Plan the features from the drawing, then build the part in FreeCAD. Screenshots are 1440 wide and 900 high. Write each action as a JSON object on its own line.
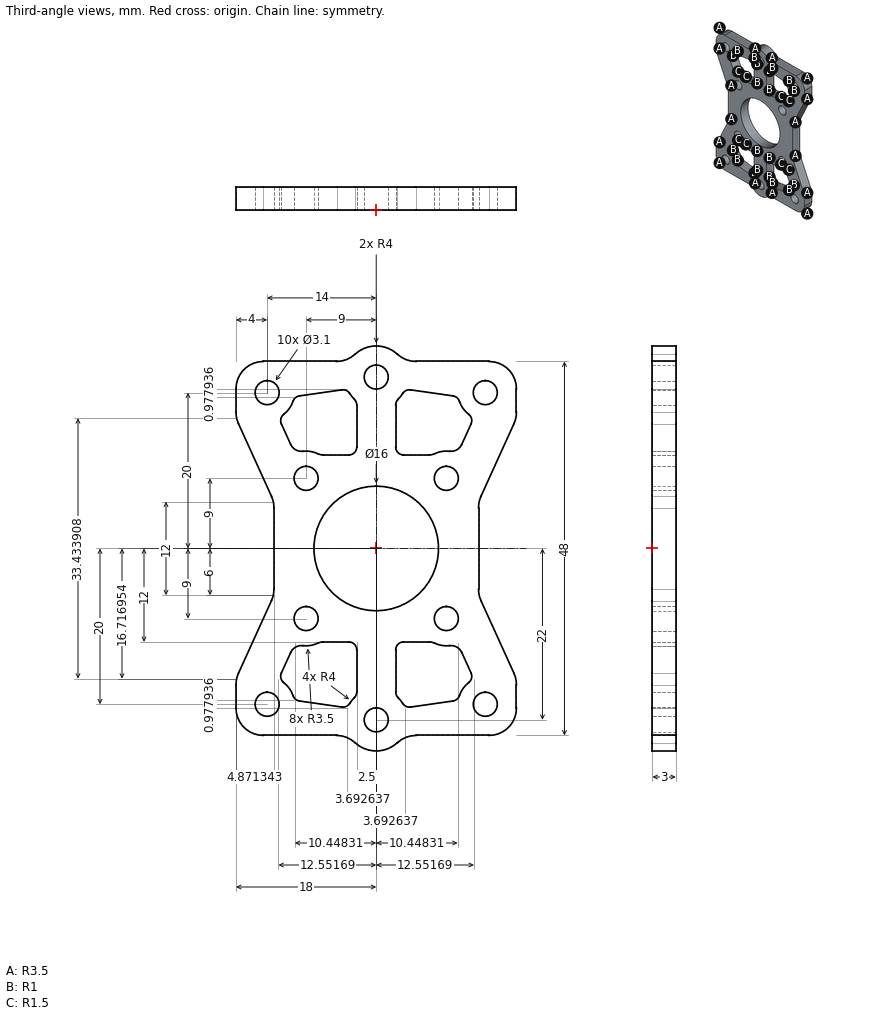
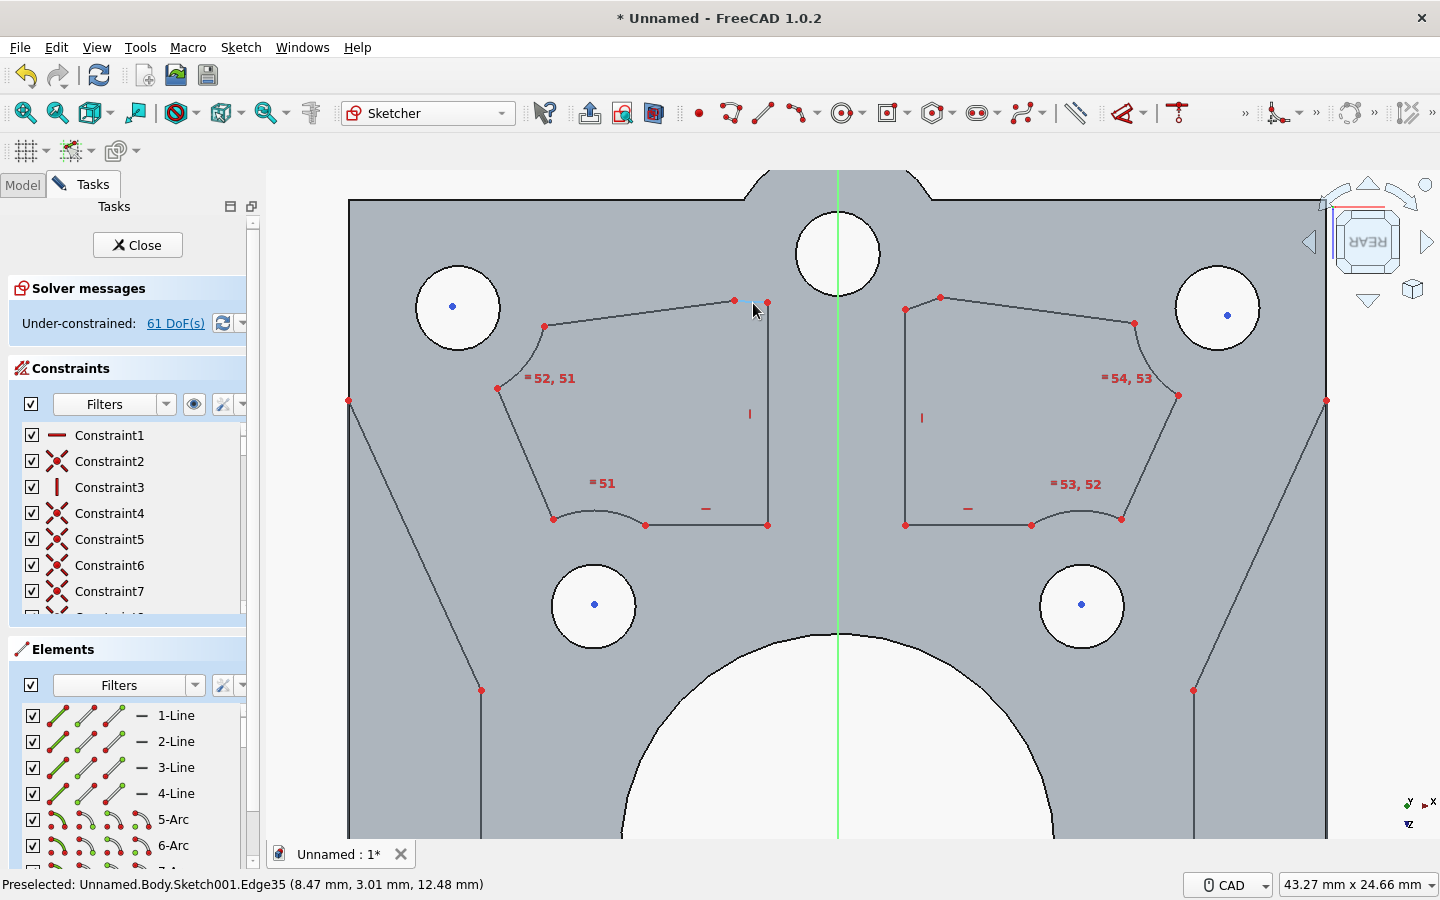
{"action": "left_click", "coordinate": [751, 302]}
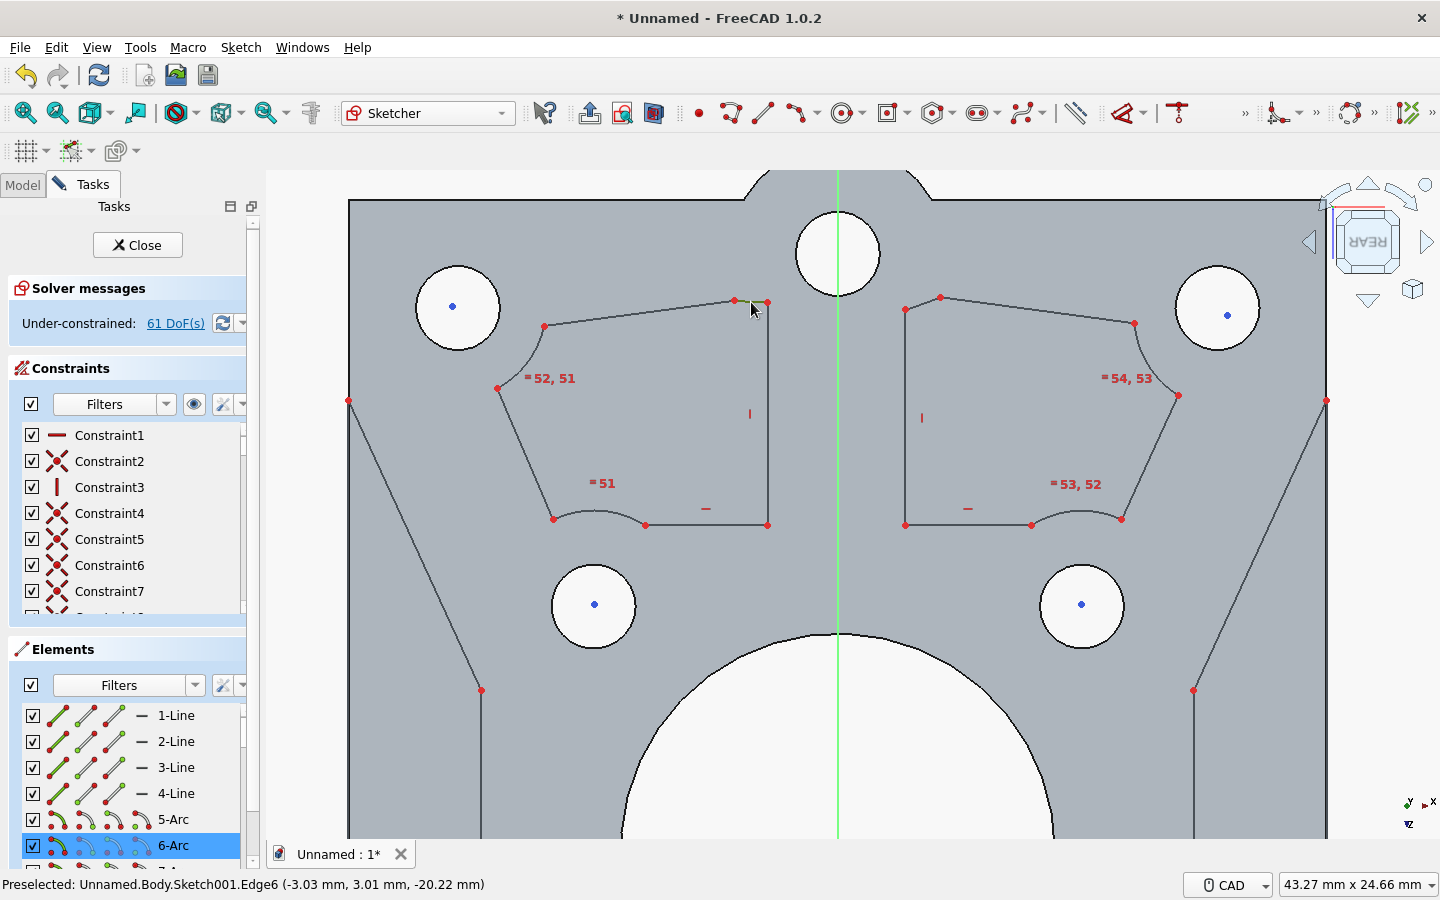
{"action": "scroll", "coordinate": [916, 306], "scroll_direction": "up", "scroll_amount": 2}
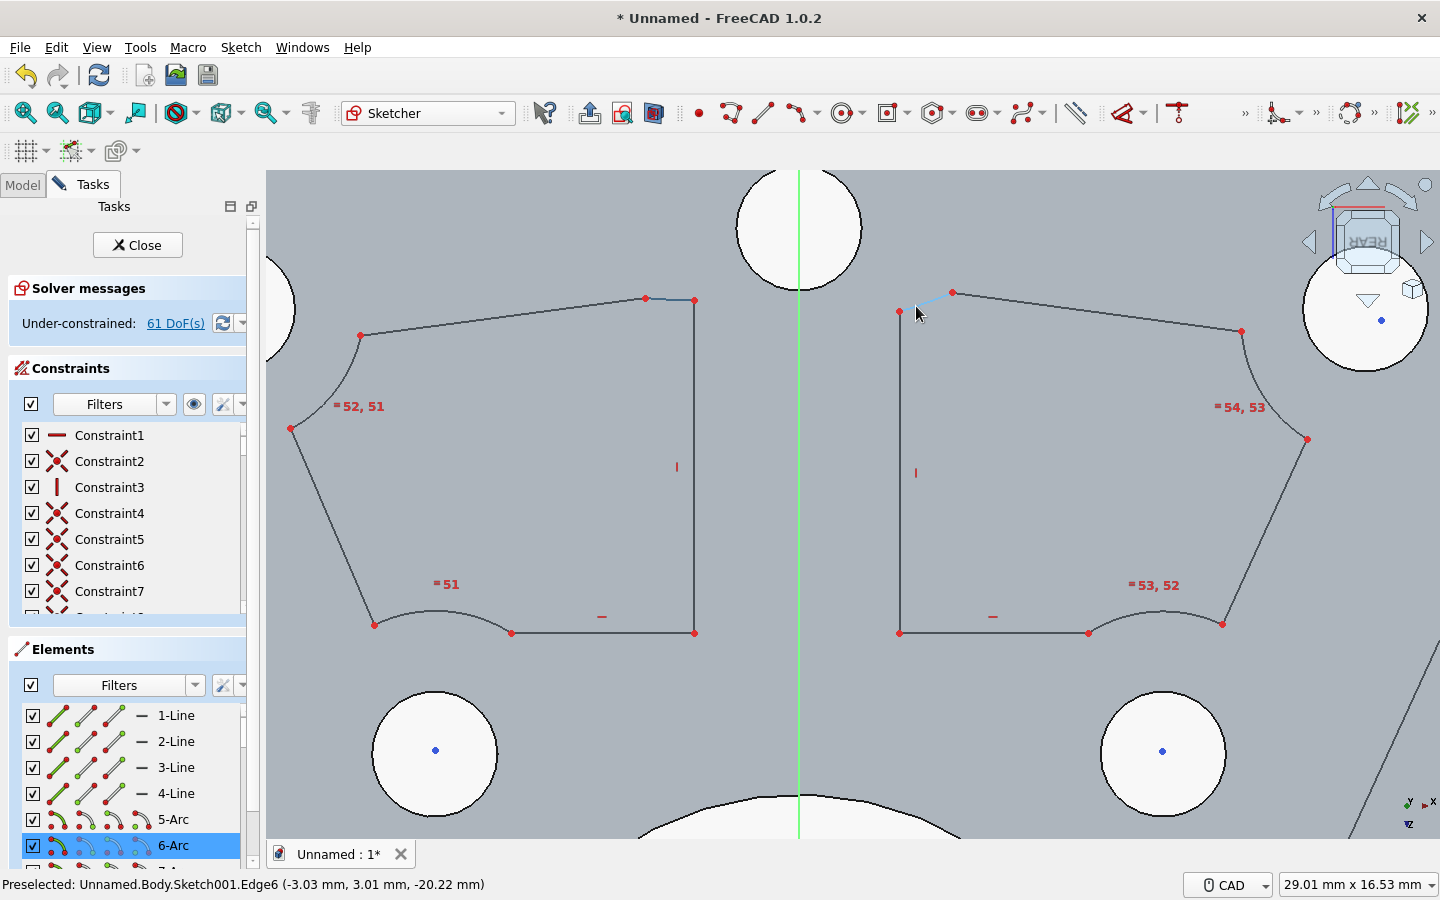
{"action": "left_click", "coordinate": [916, 306]}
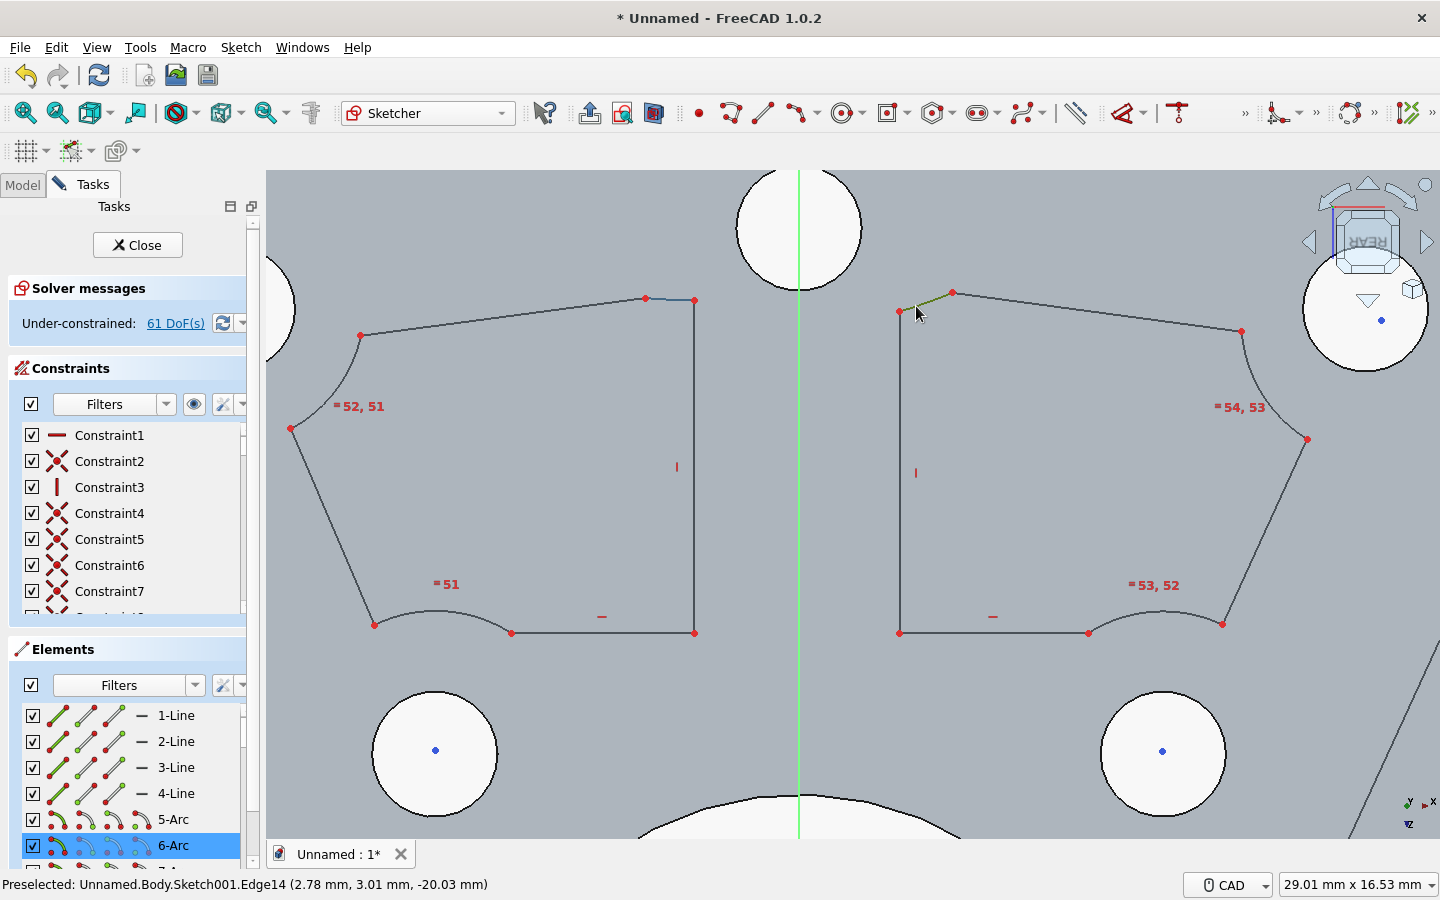
{"action": "scroll", "coordinate": [780, 304], "scroll_direction": "down", "scroll_amount": 7}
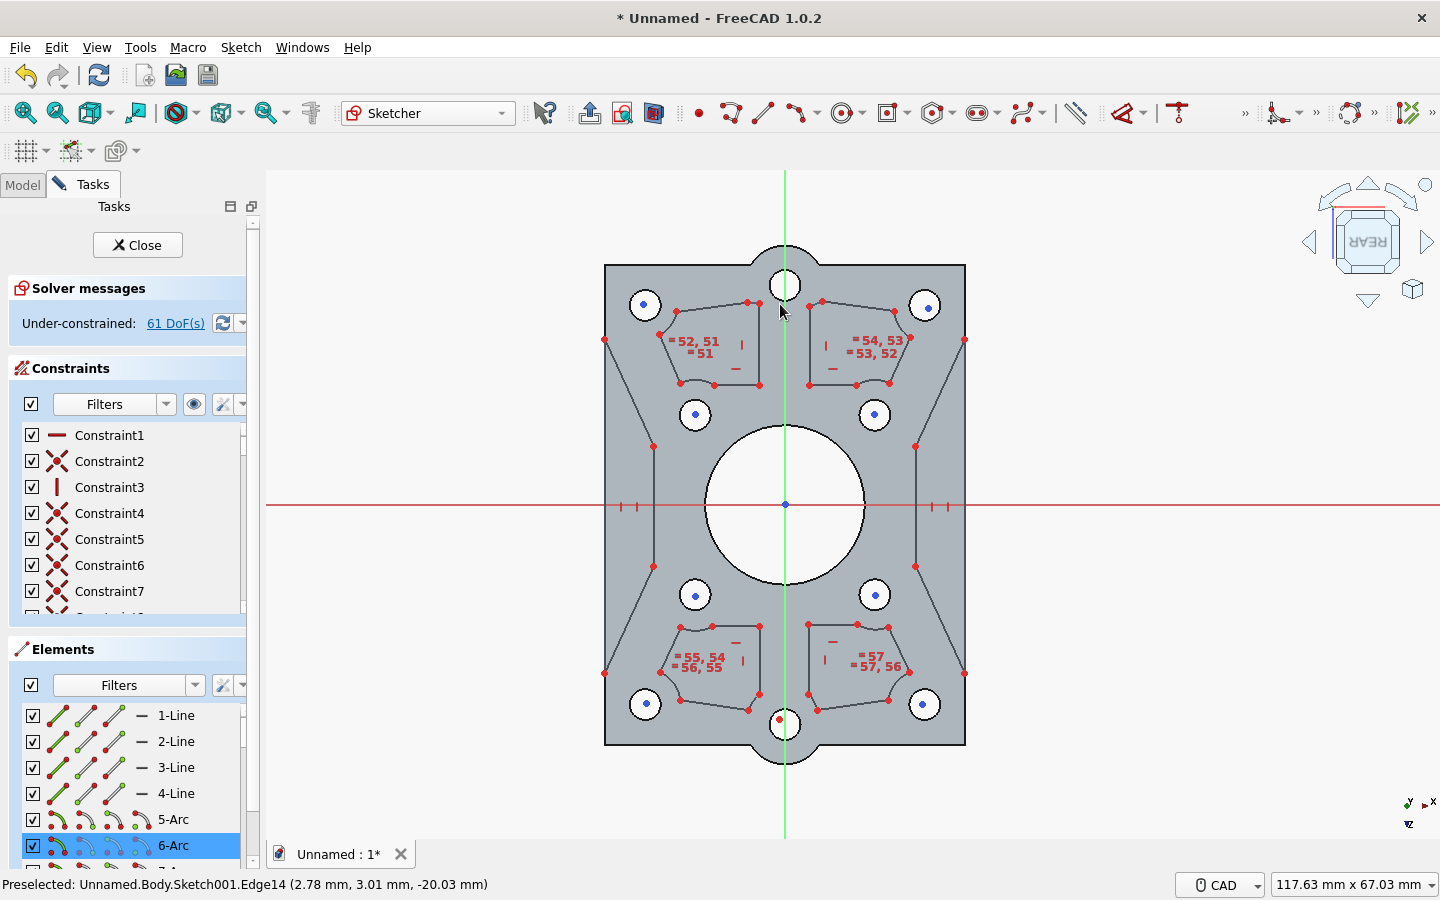
{"action": "scroll", "coordinate": [756, 698], "scroll_direction": "up", "scroll_amount": 5}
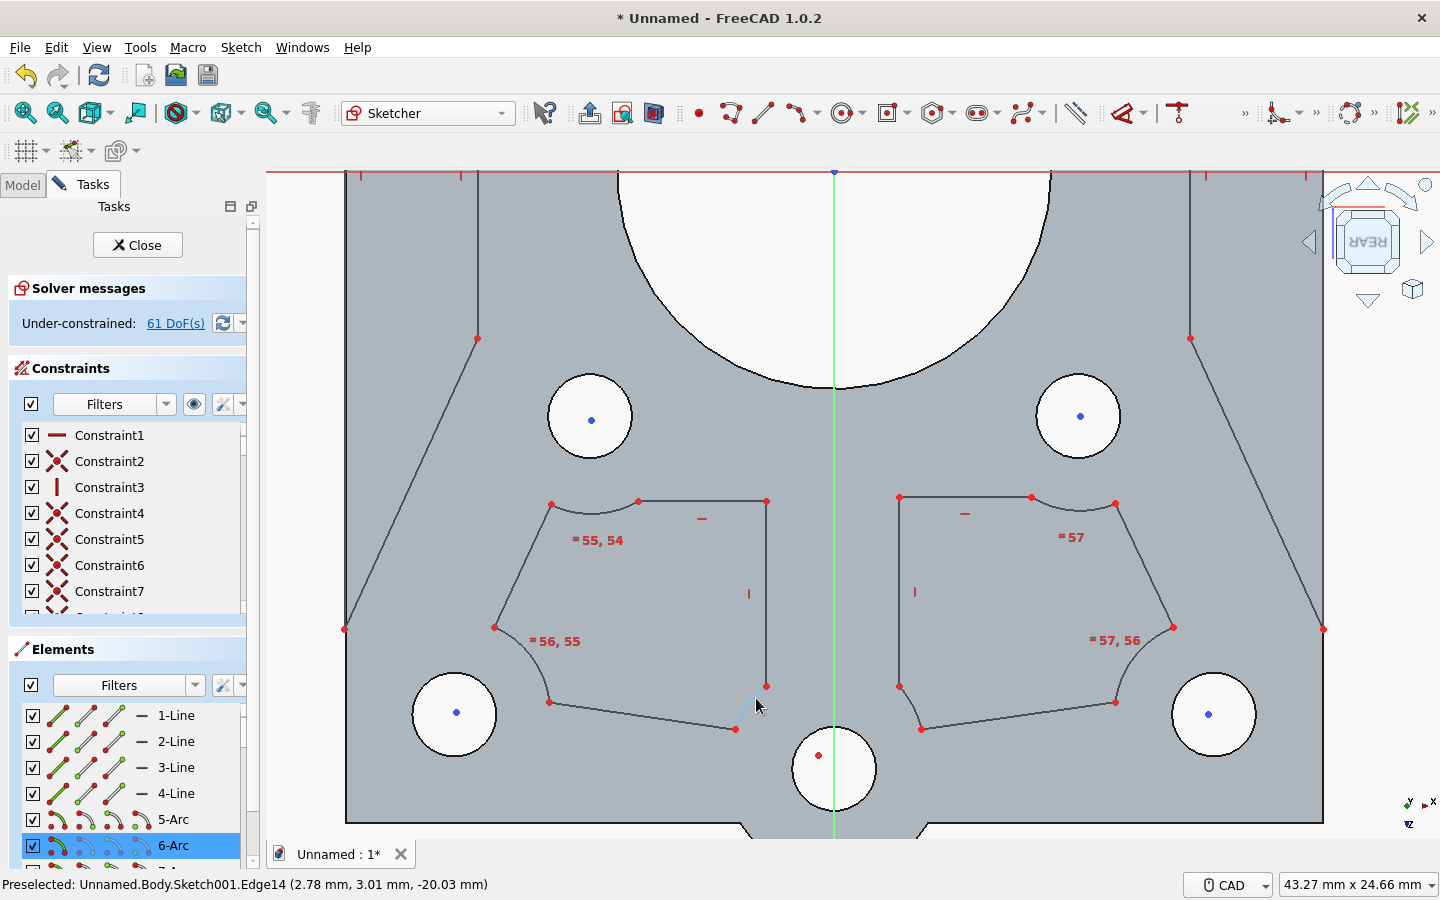
{"action": "left_click", "coordinate": [754, 697]}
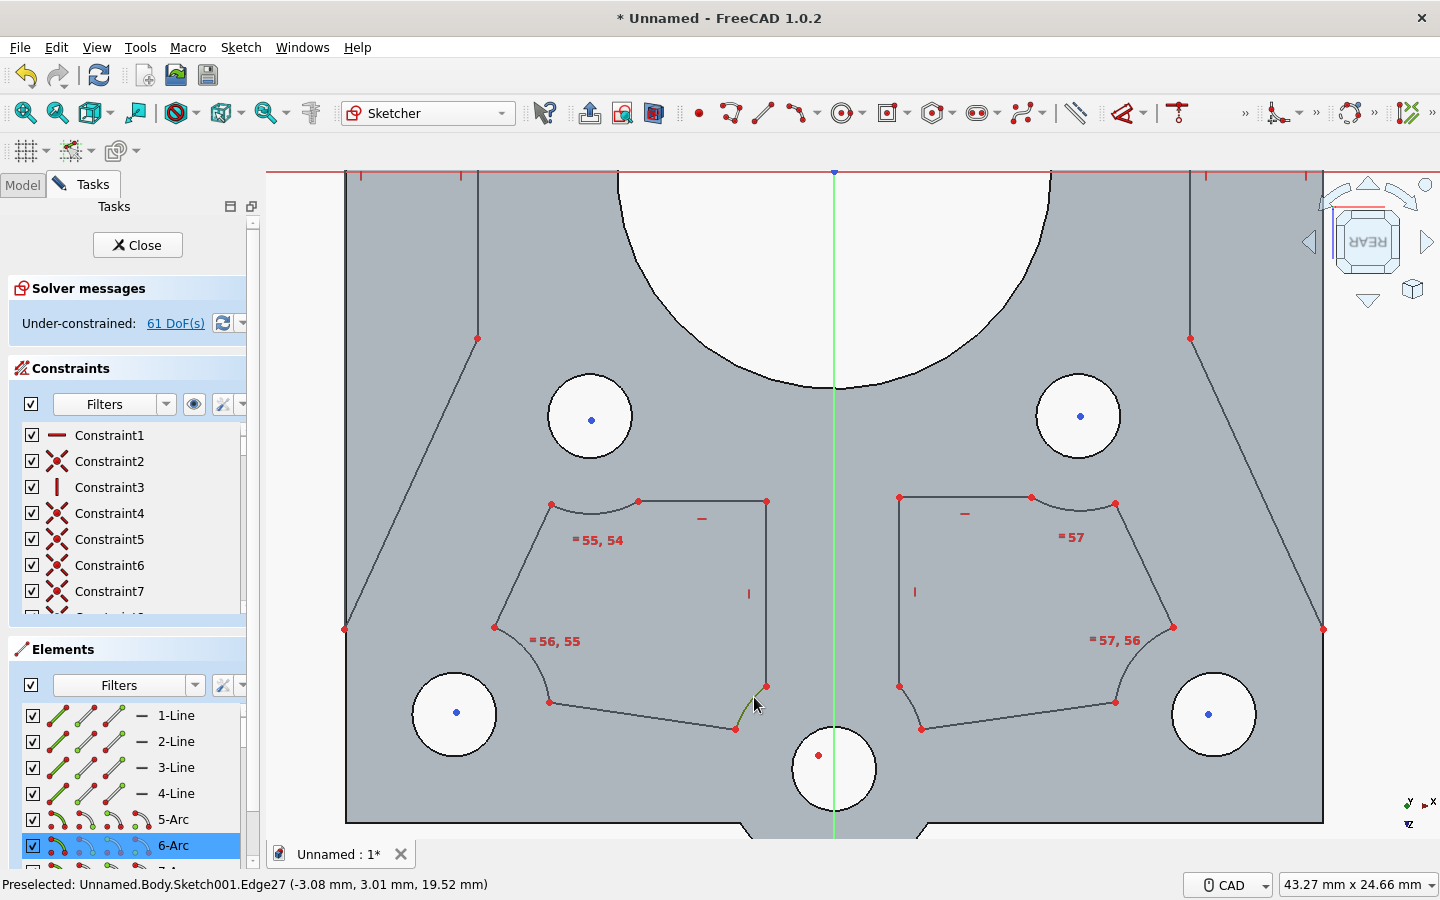
{"action": "left_click", "coordinate": [917, 715]}